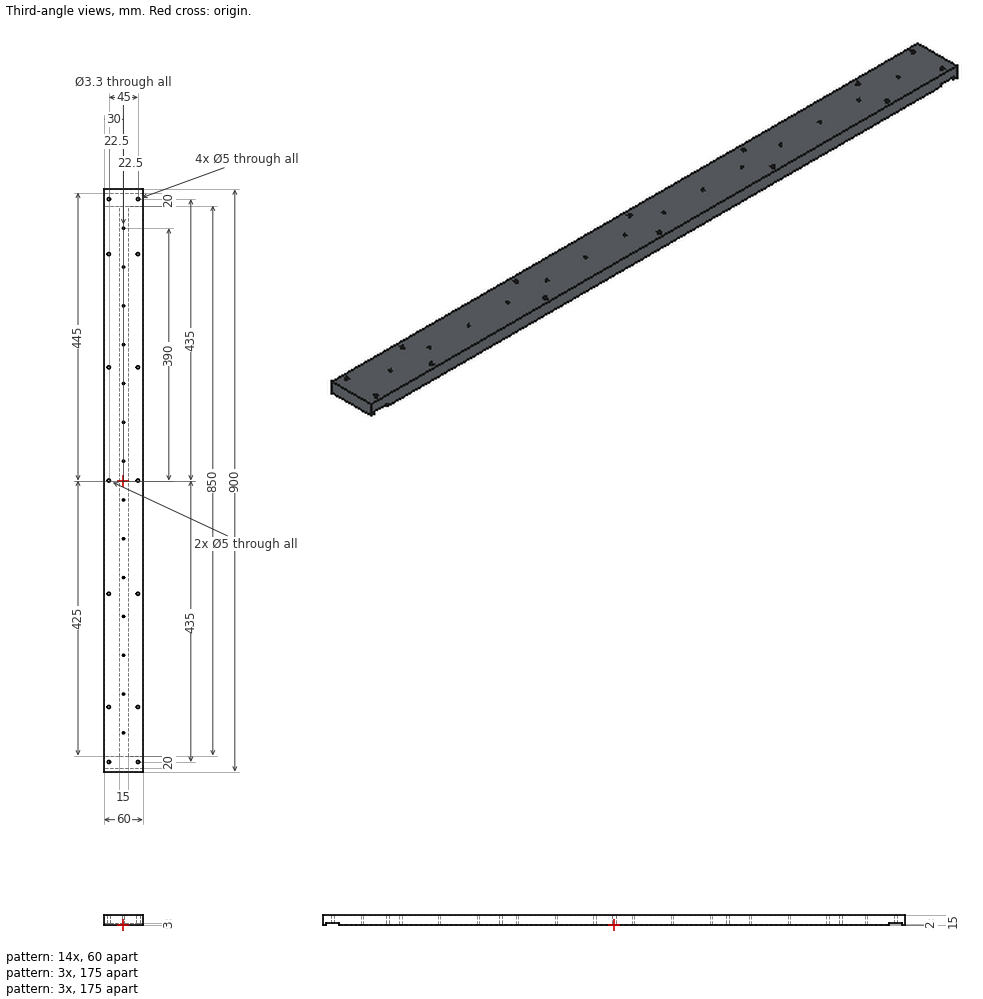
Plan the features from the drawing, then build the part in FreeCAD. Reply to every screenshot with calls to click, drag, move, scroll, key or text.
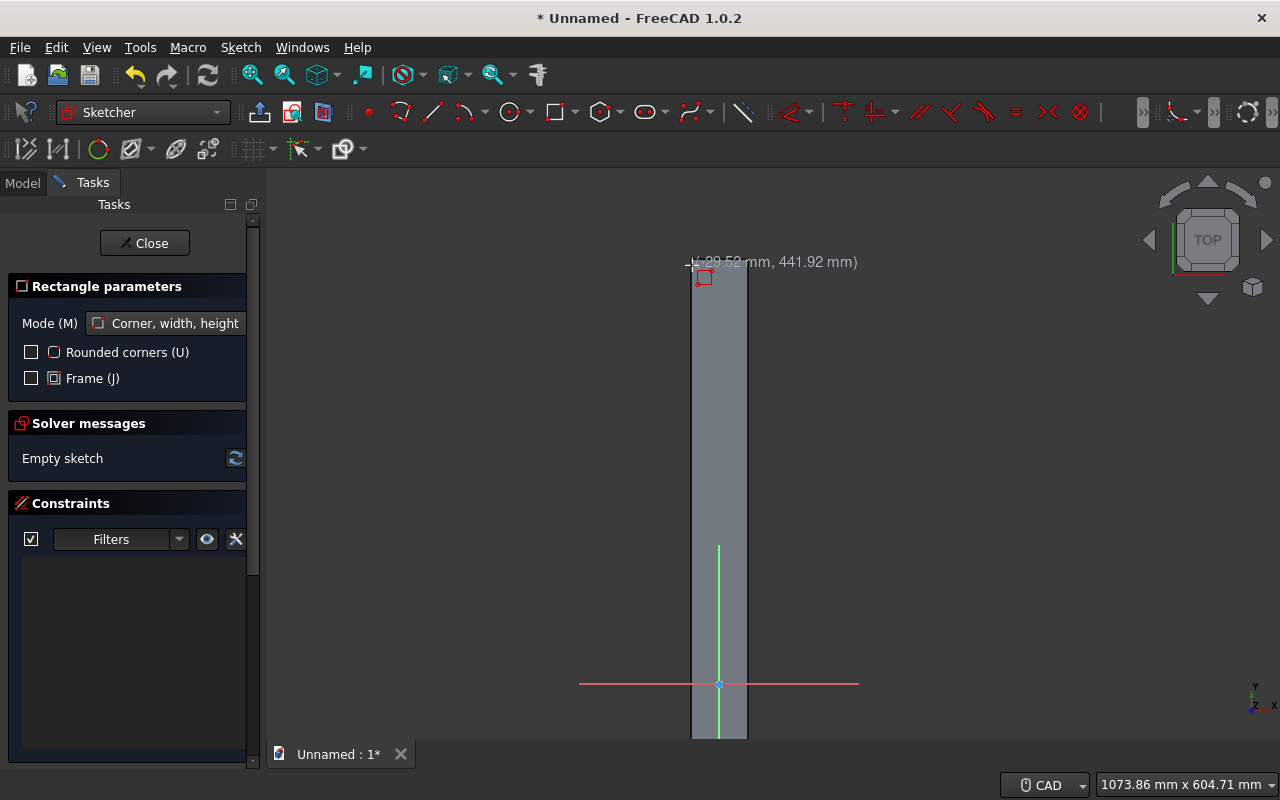
click(691, 264)
move(748, 283)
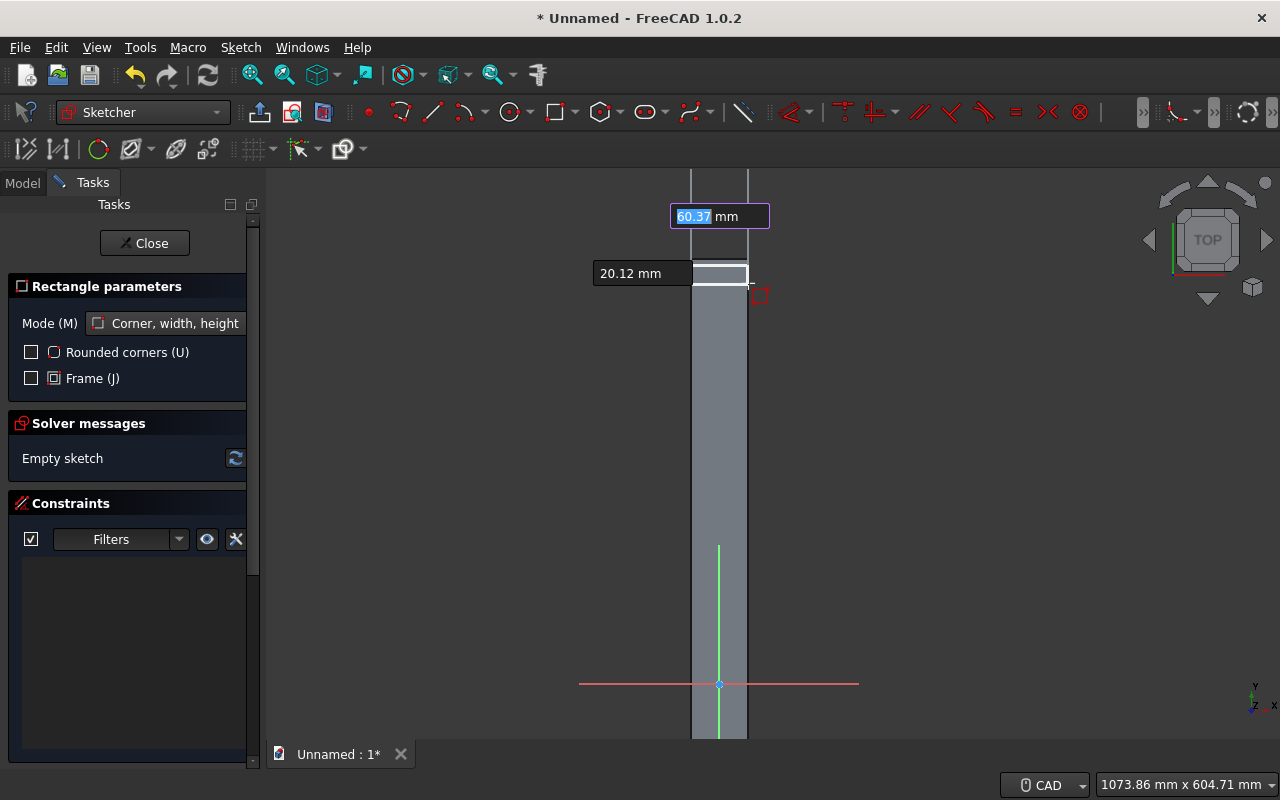
text(60)
key(Tab)
text(20)
key(Return)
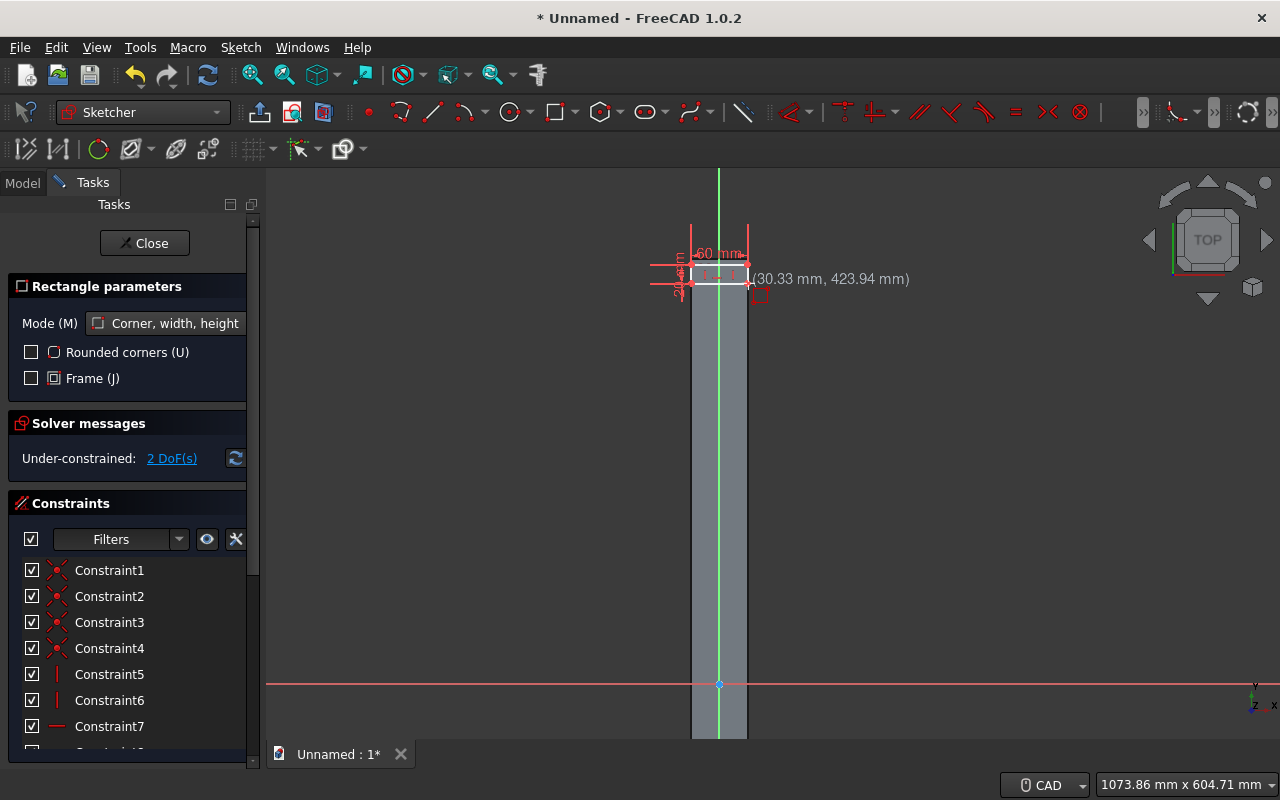
scroll(692, 265, down, 4)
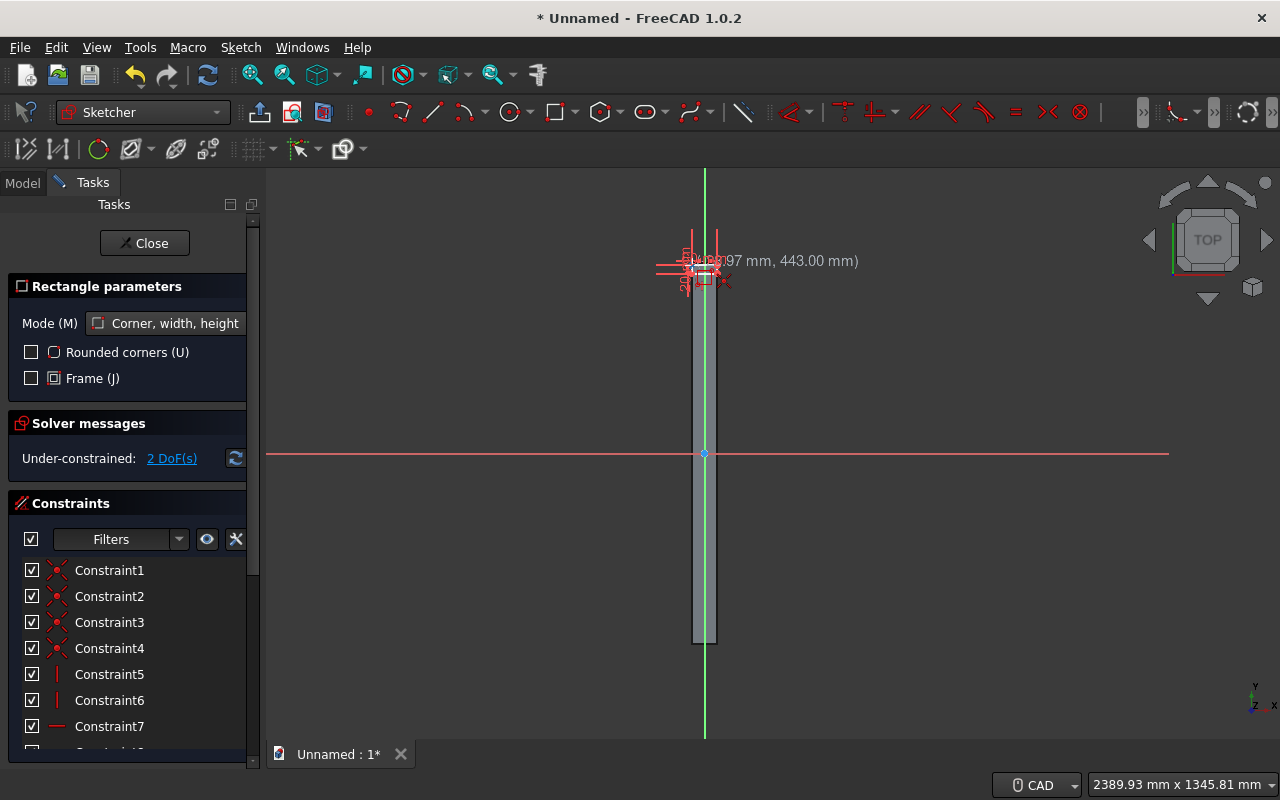
scroll(692, 634, up, 4)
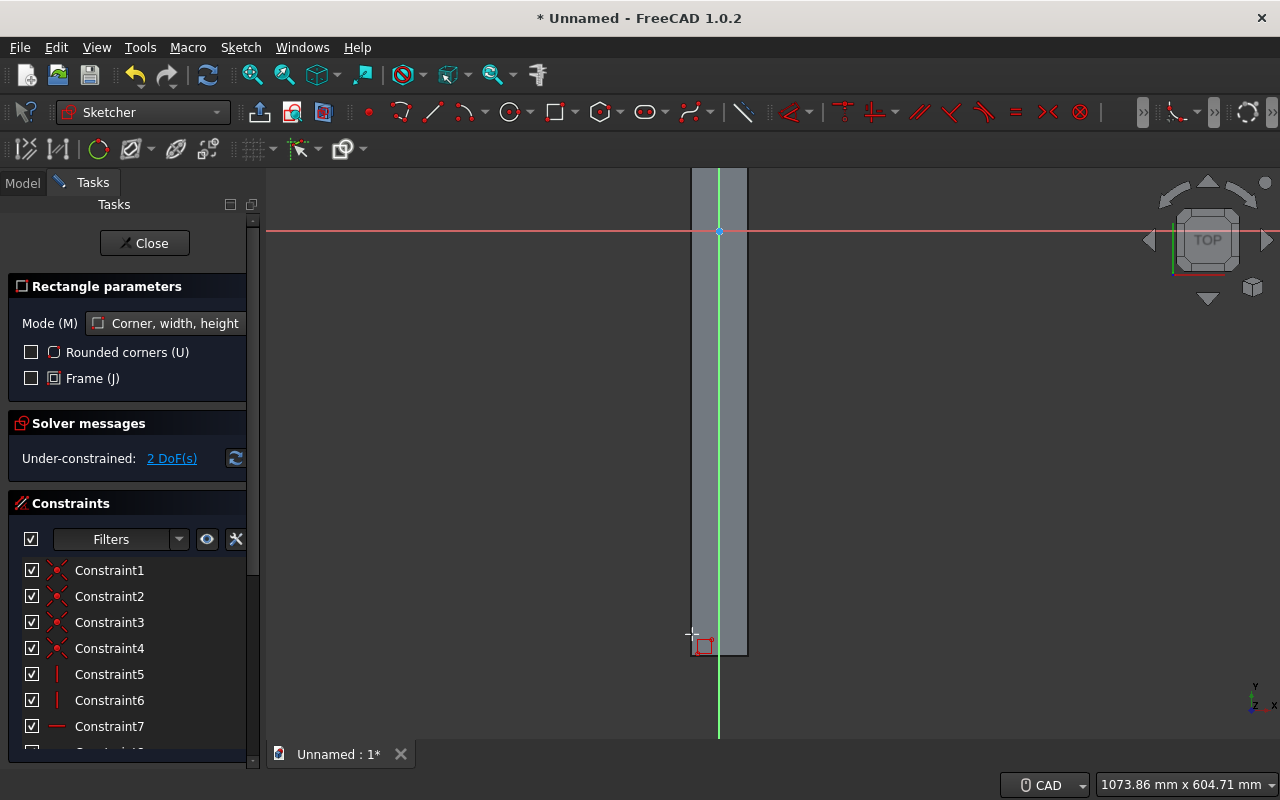
click(691, 633)
move(748, 651)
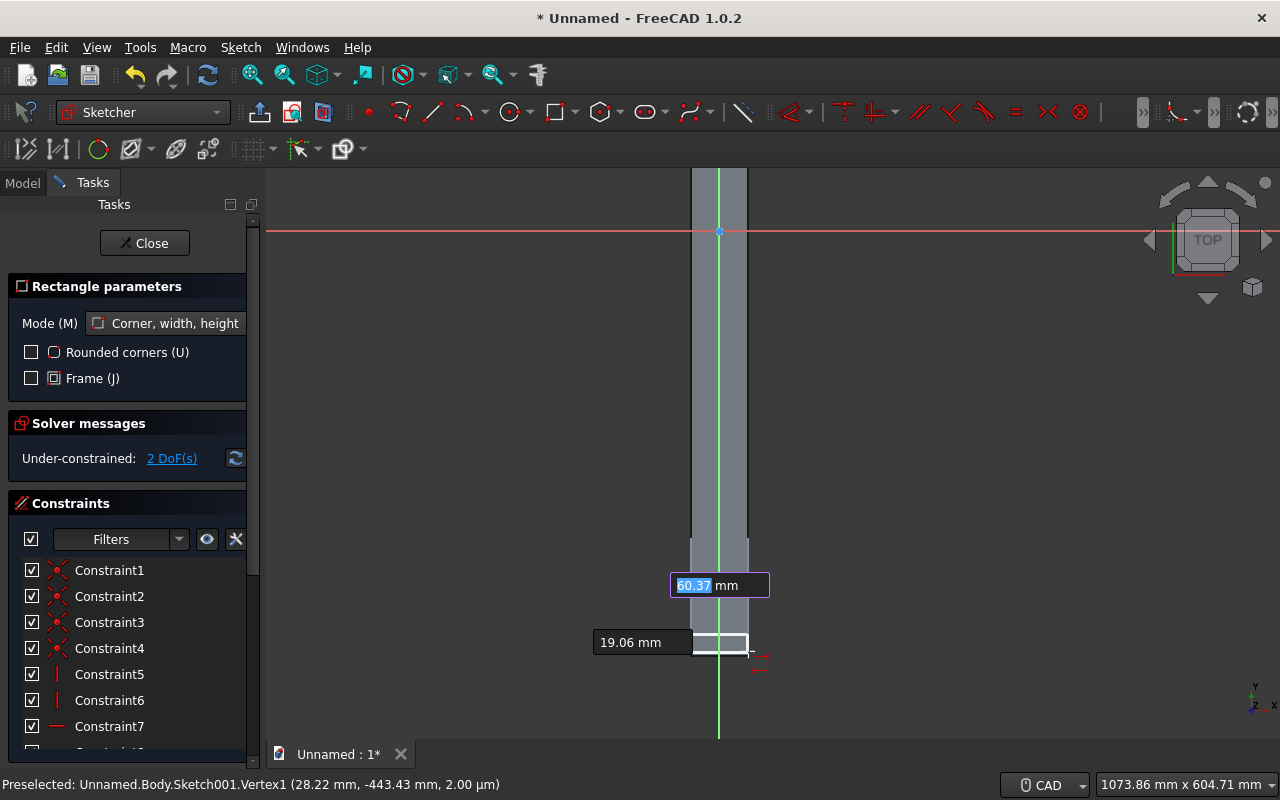
text(60)
key(Tab)
text(20)
key(Return)
key(Escape)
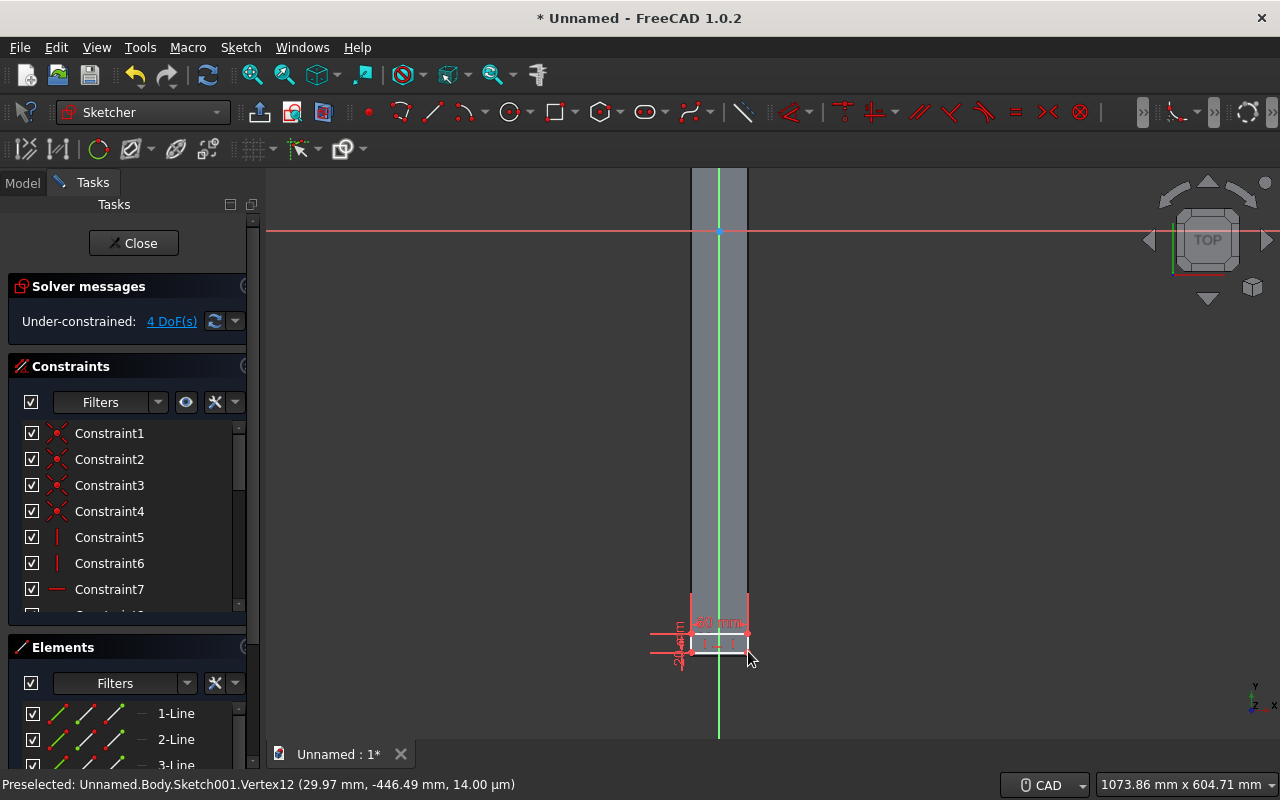
click(790, 112)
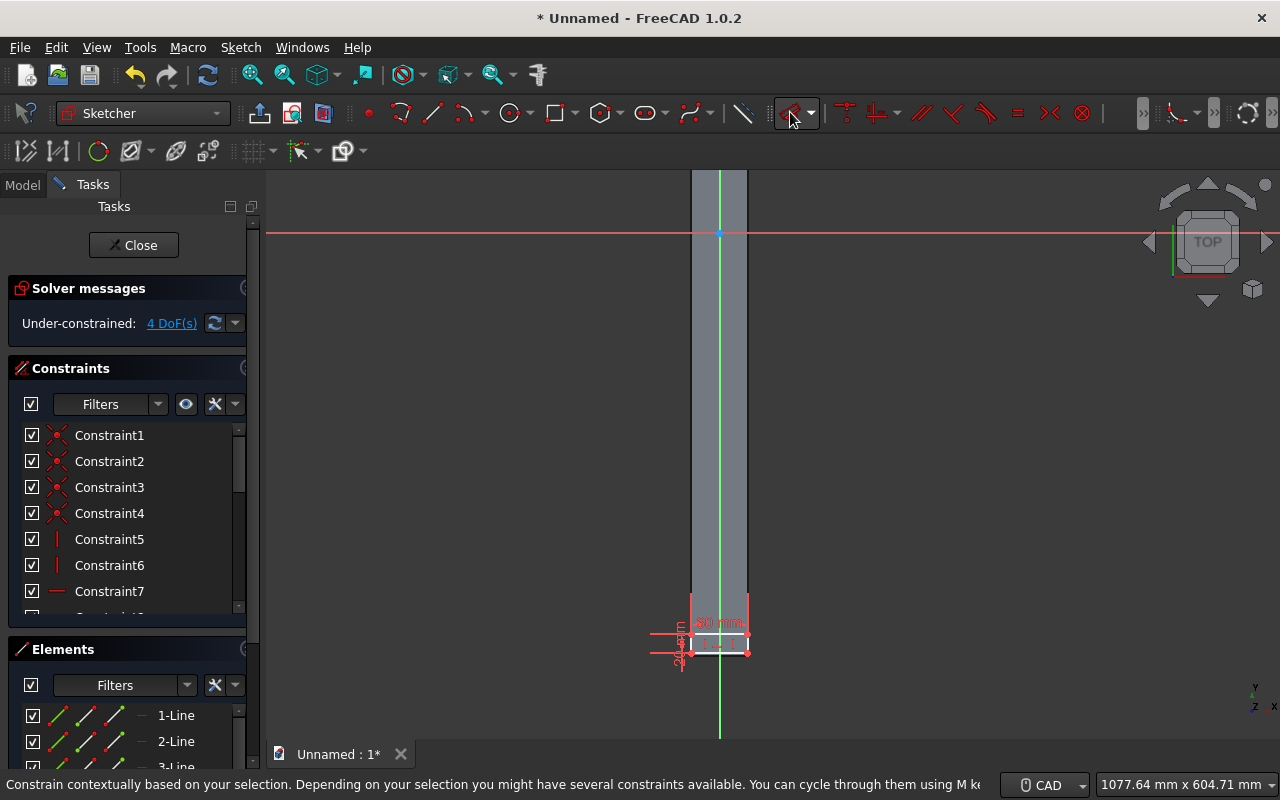
scroll(692, 635, down, 4)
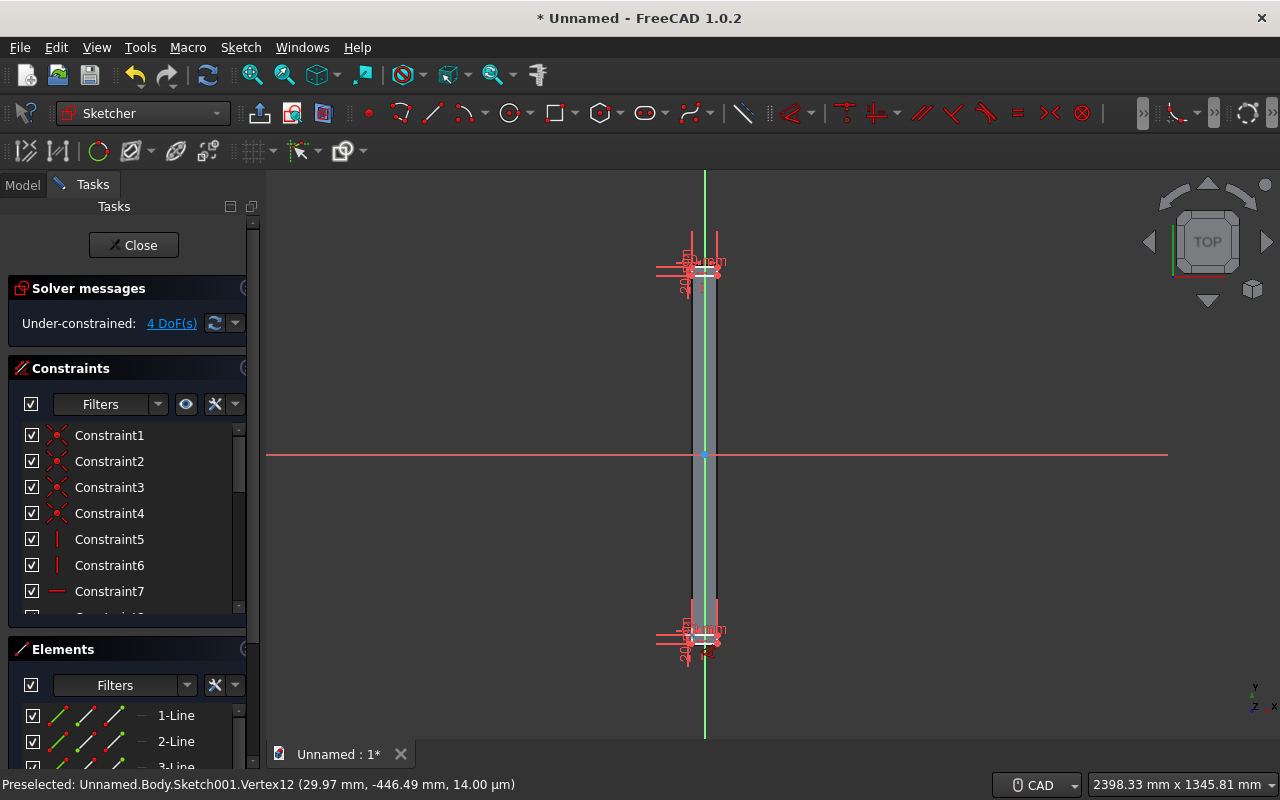
scroll(692, 267, up, 6)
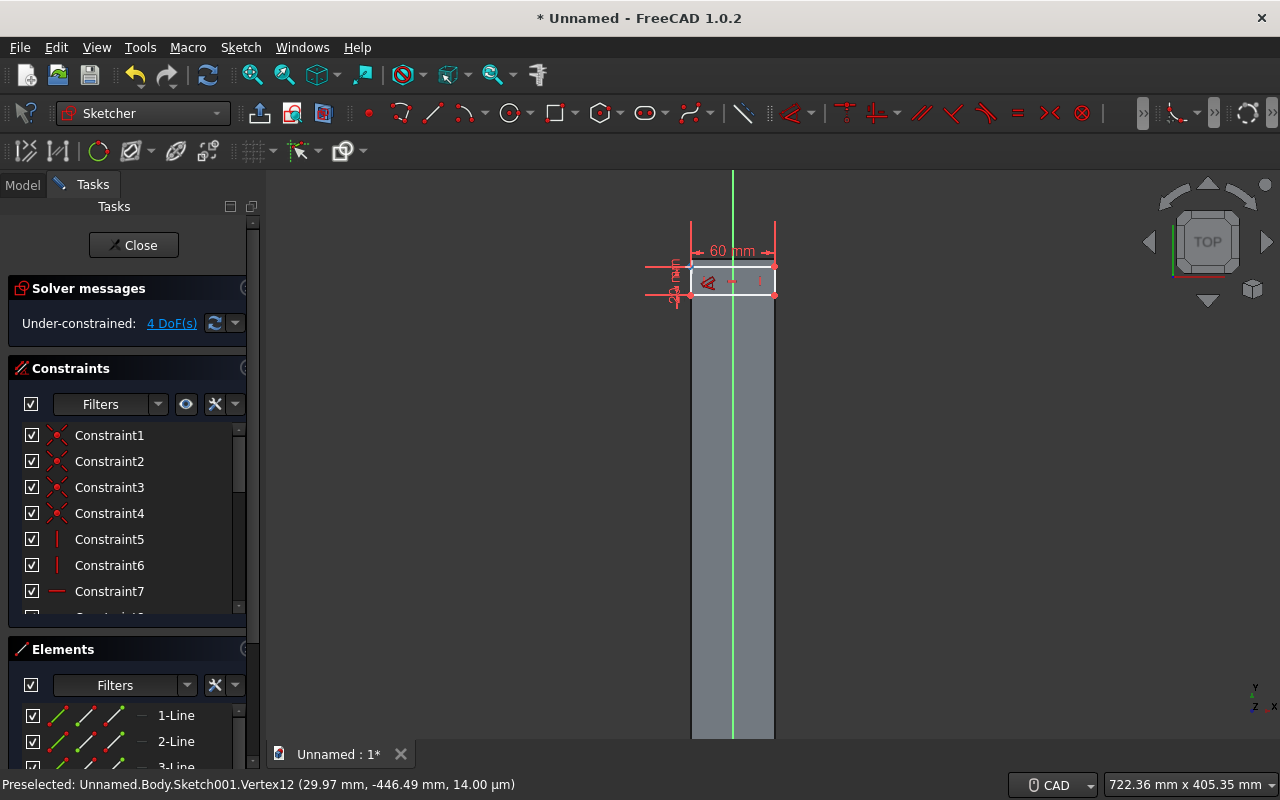
click(691, 267)
click(712, 233)